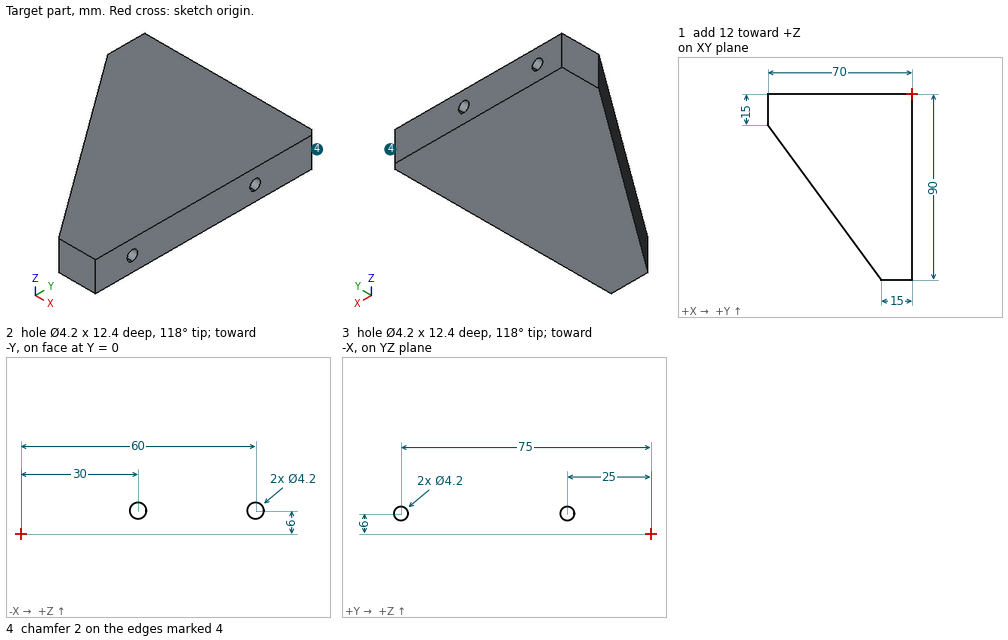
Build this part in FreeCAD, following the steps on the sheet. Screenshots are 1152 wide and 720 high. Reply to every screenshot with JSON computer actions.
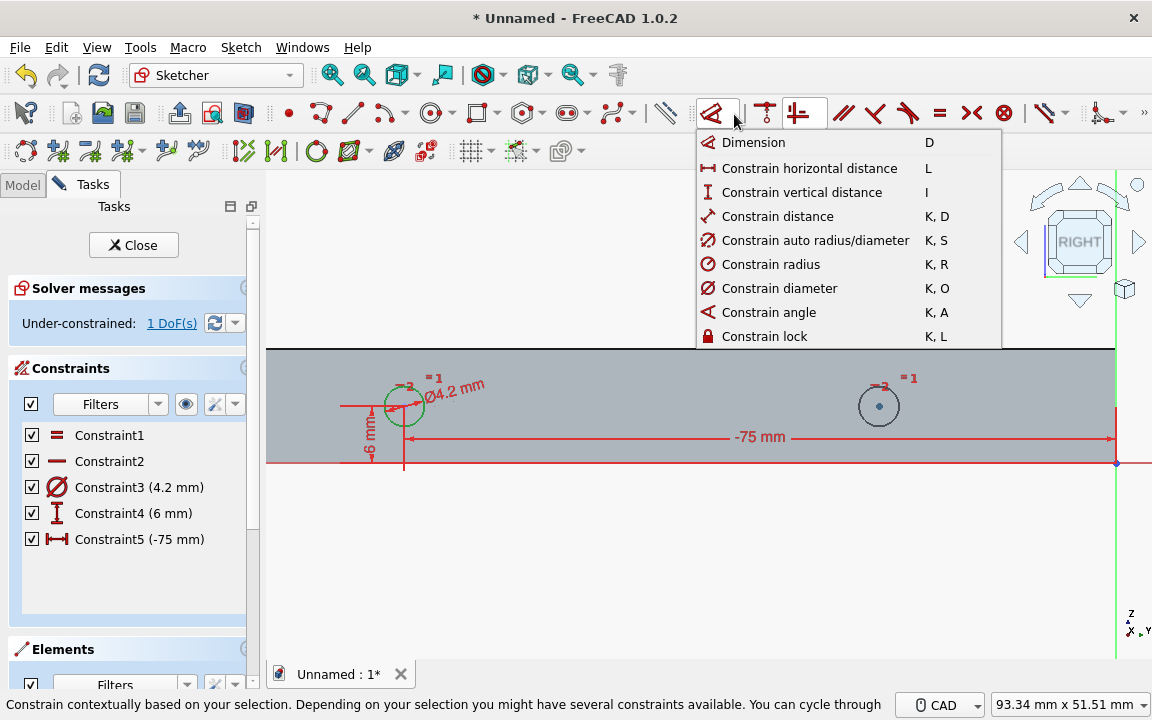
{"action": "left_click", "coordinate": [849, 168]}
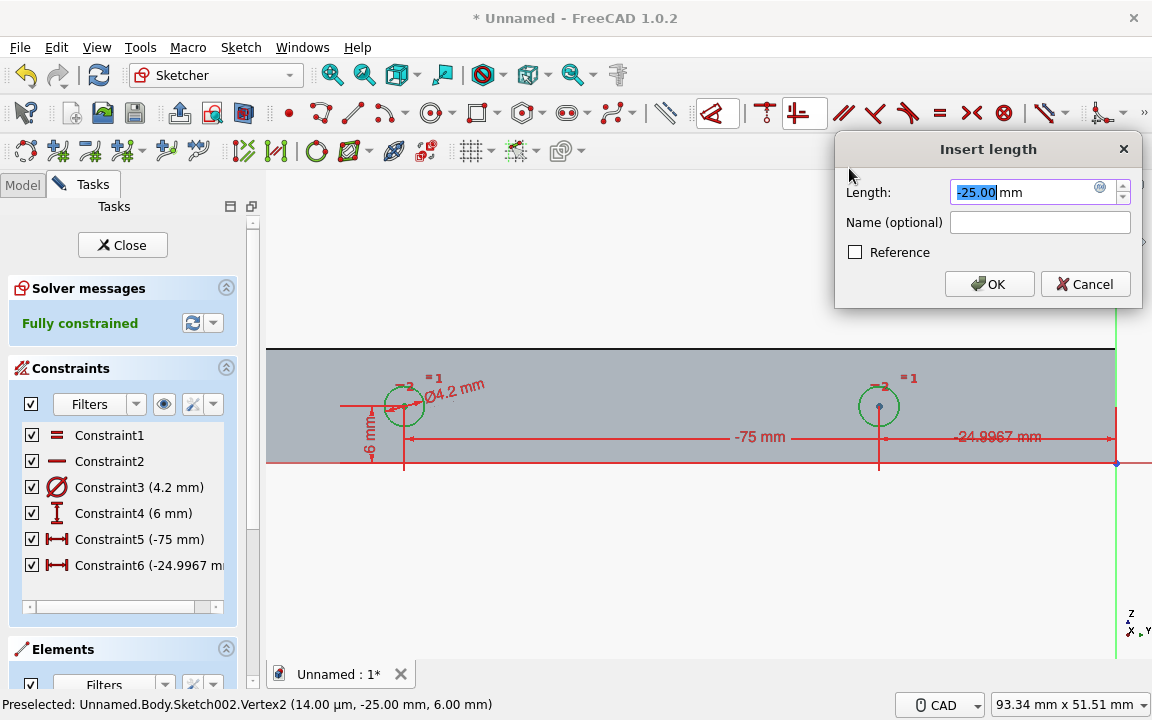
{"action": "type", "text": "-25"}
{"action": "key", "text": "Return"}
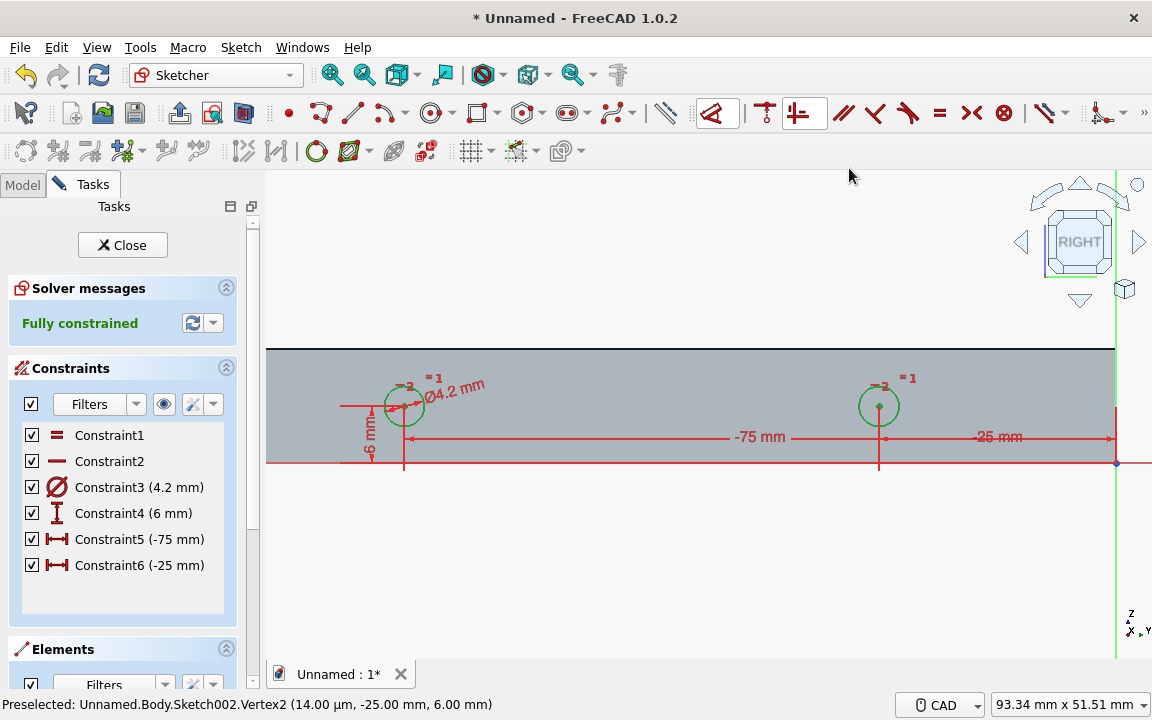
{"action": "left_click", "coordinate": [123, 245]}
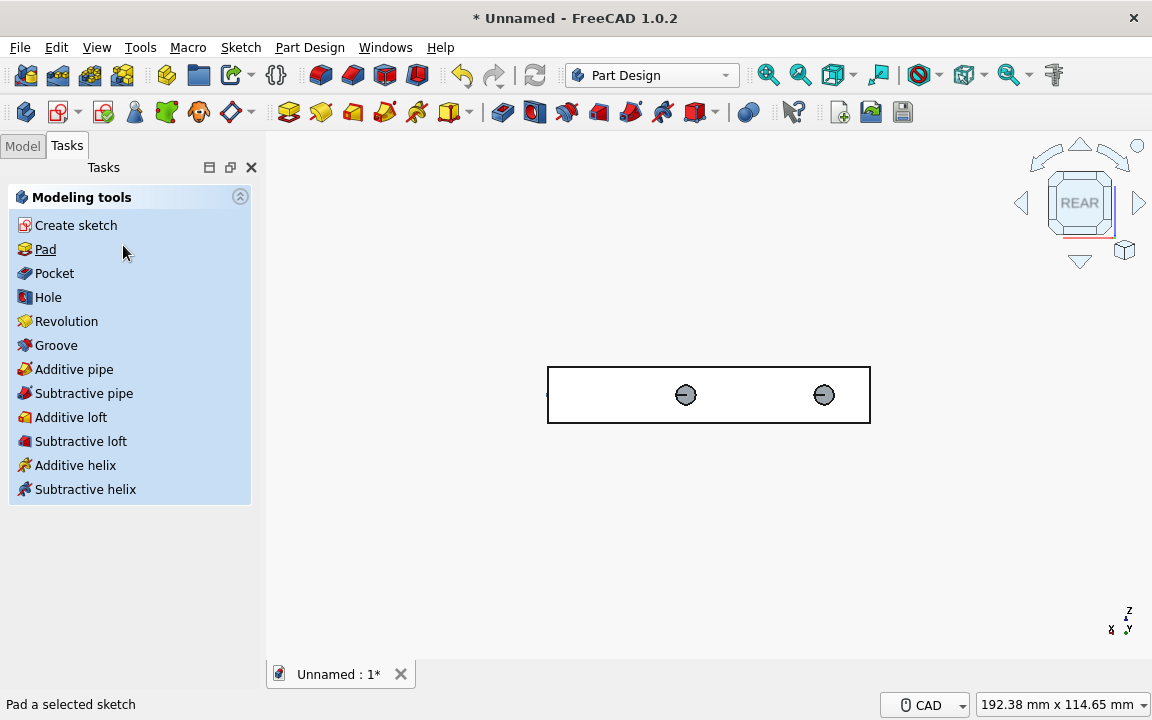
{"action": "left_click", "coordinate": [536, 112]}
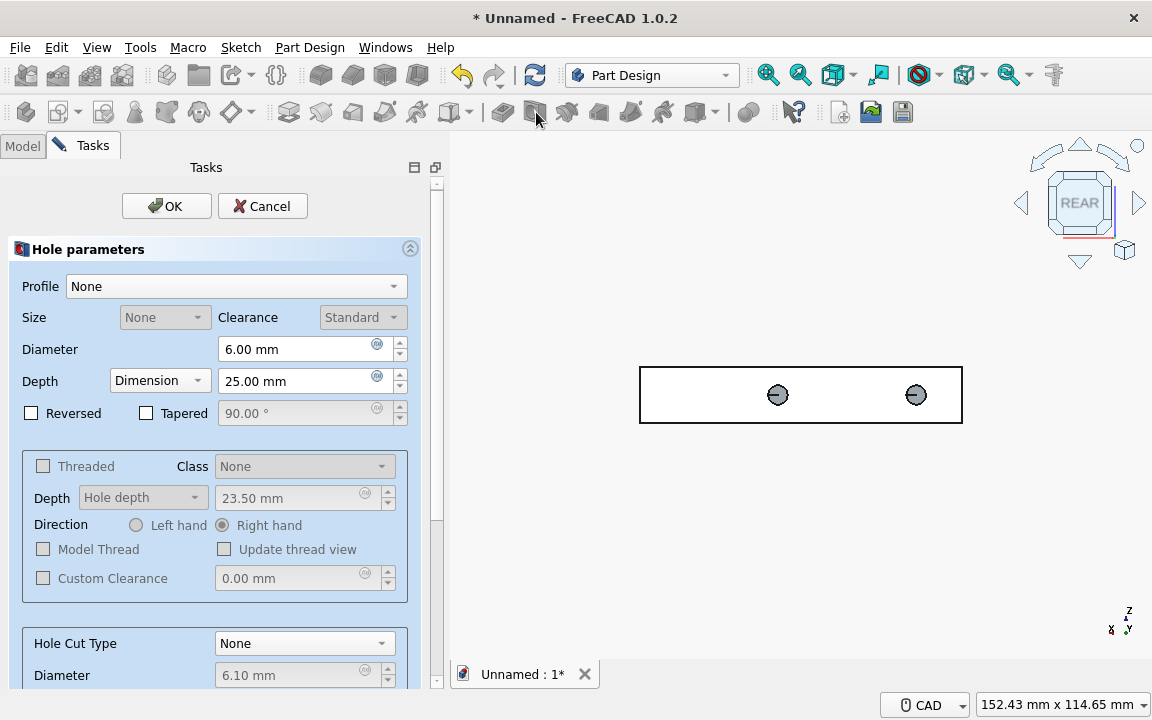
{"action": "triple_click", "coordinate": [305, 349]}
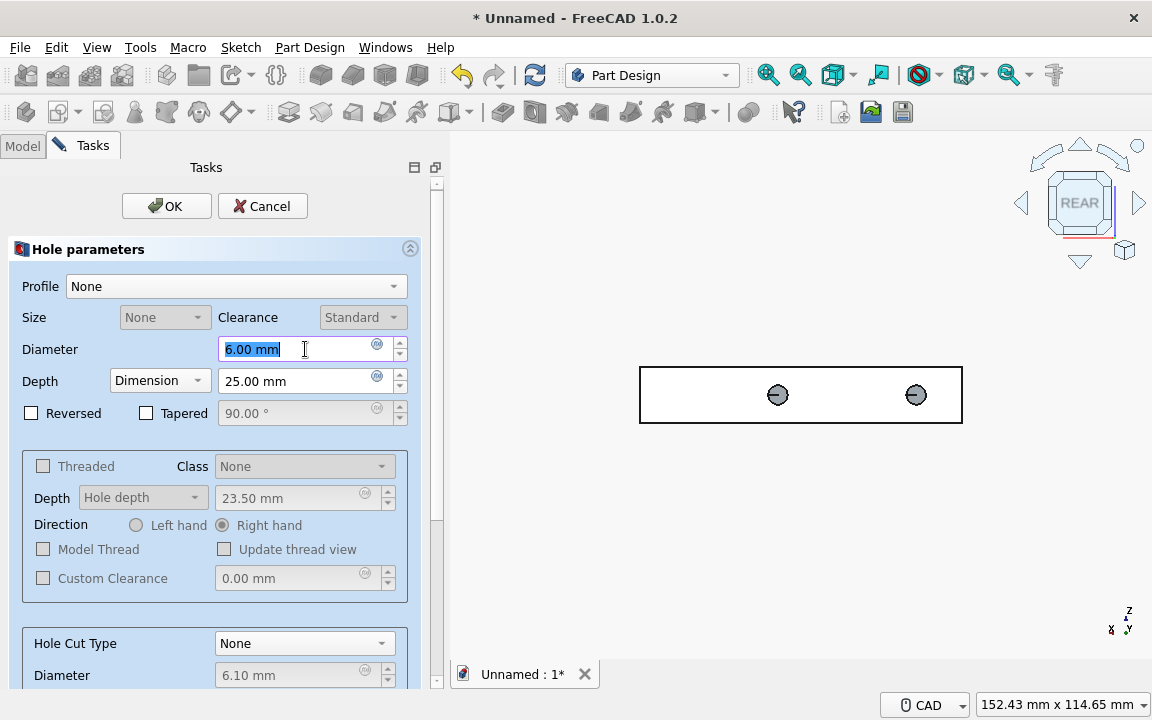
{"action": "type", "text": "4.2"}
{"action": "key", "text": "Tab"}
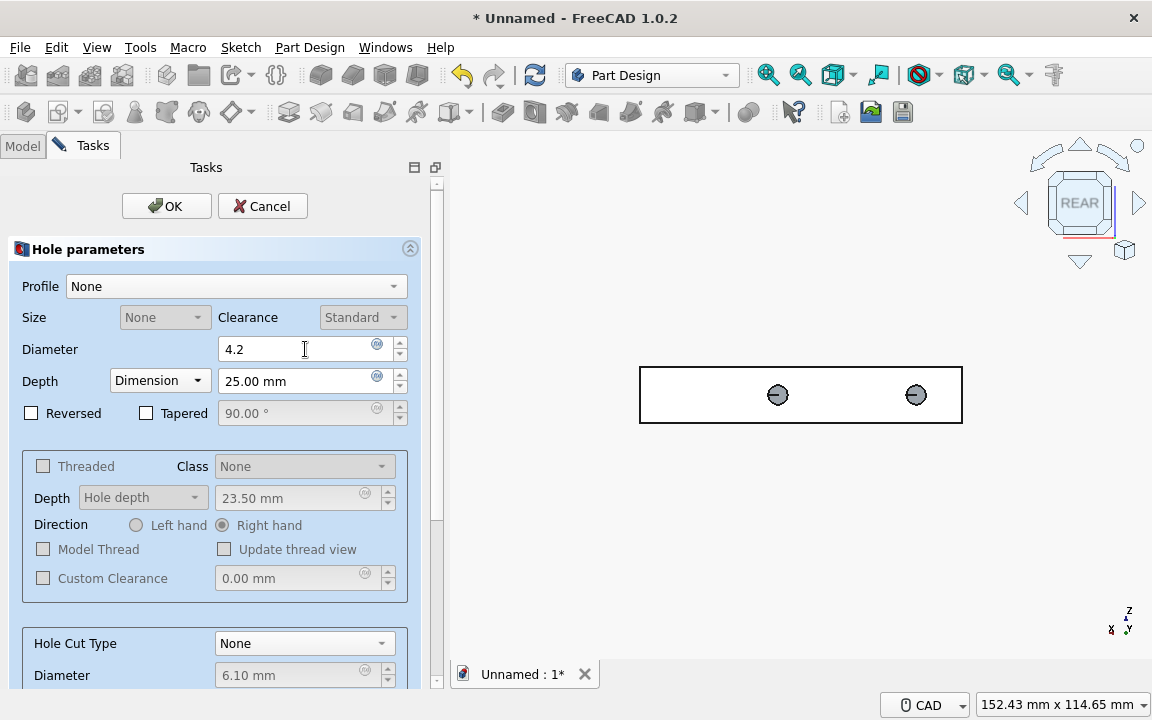
{"action": "triple_click", "coordinate": [305, 381]}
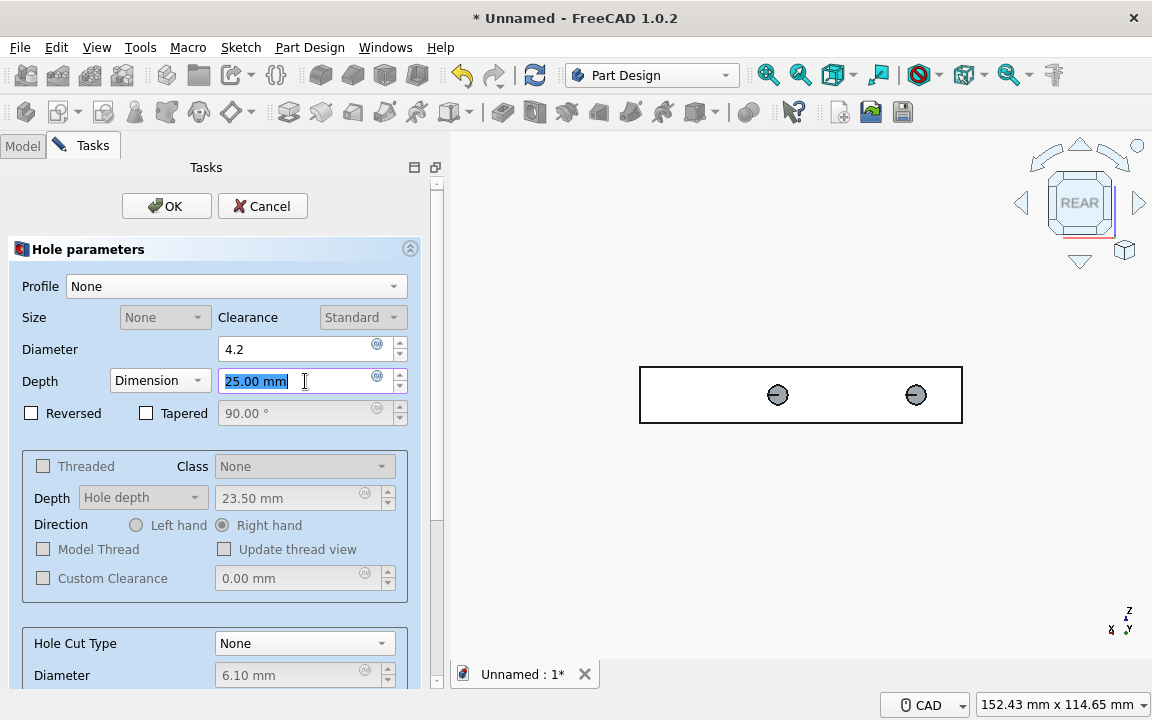
{"action": "type", "text": "12.4"}
{"action": "key", "text": "Tab"}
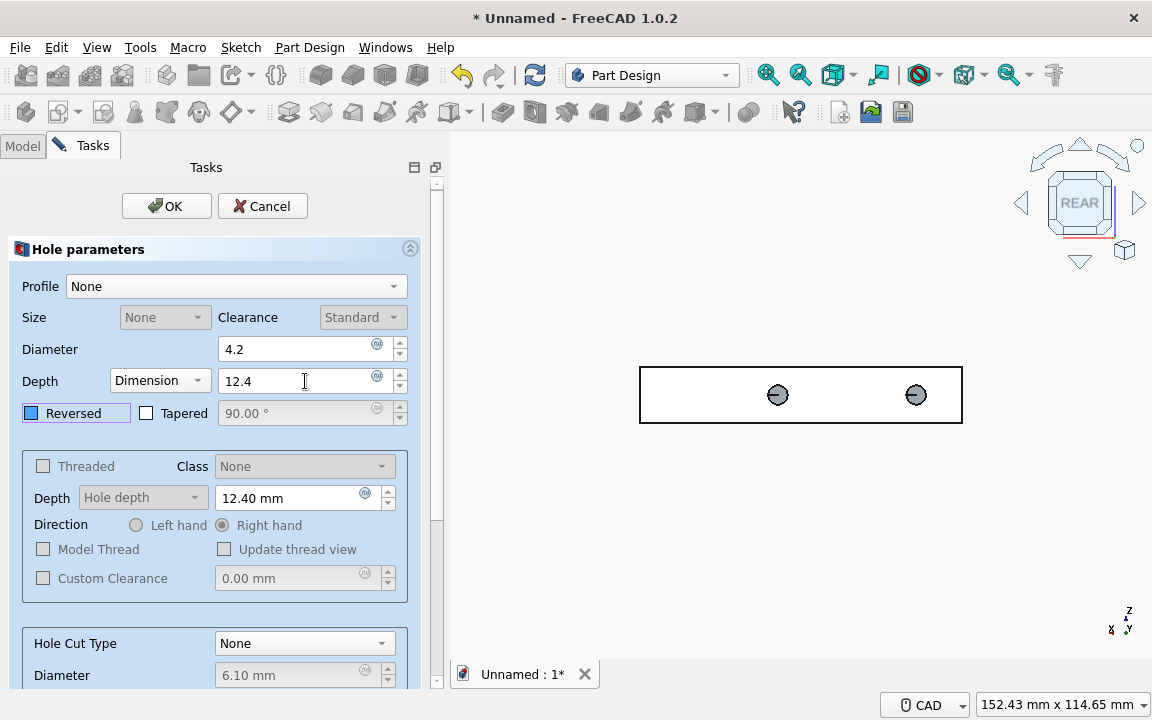
{"action": "left_click", "coordinate": [167, 206]}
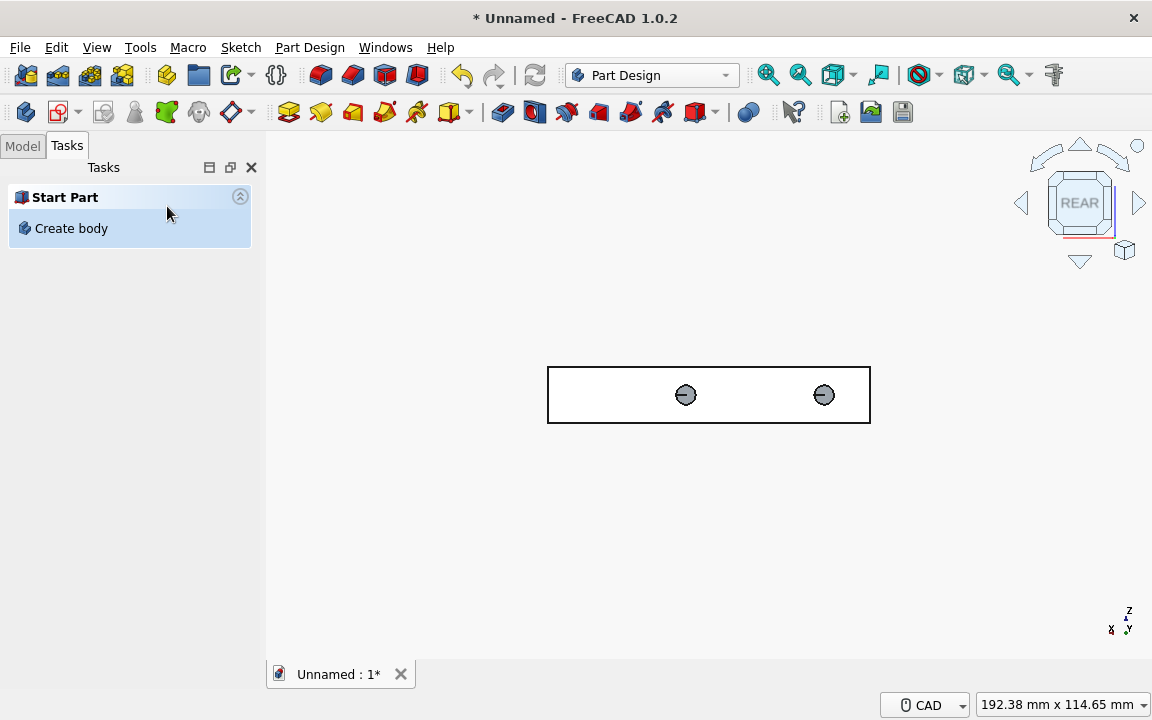
{"action": "key", "text": "v f"}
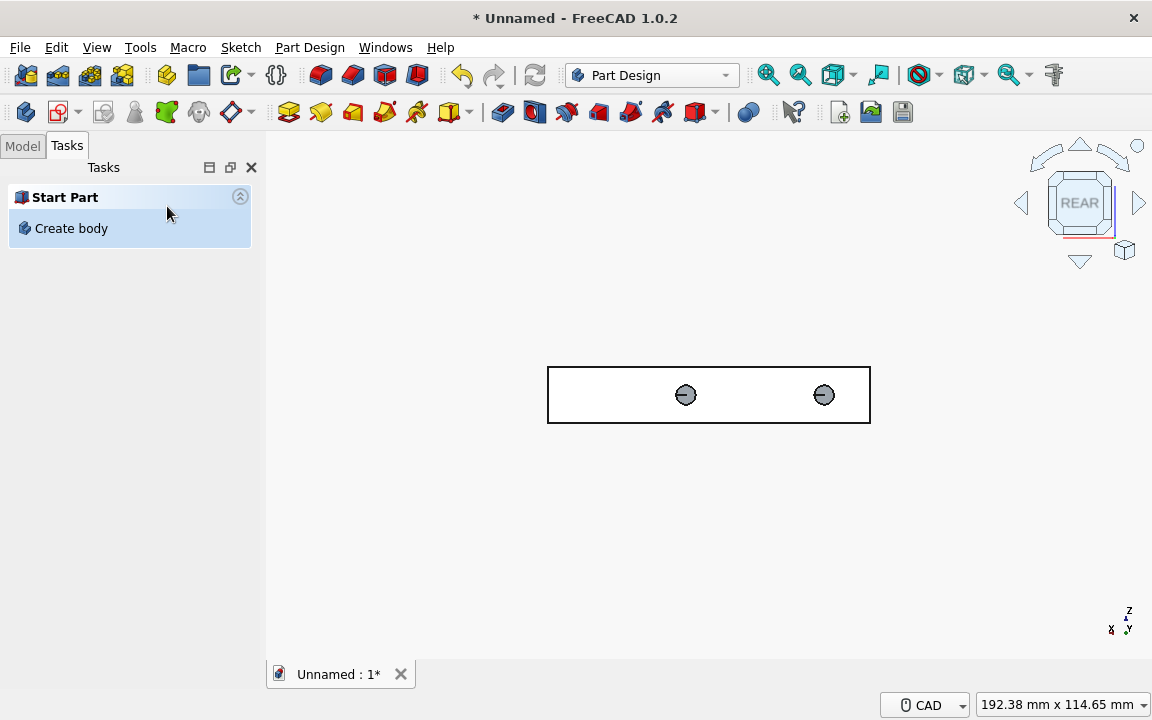
{"action": "key", "text": "0"}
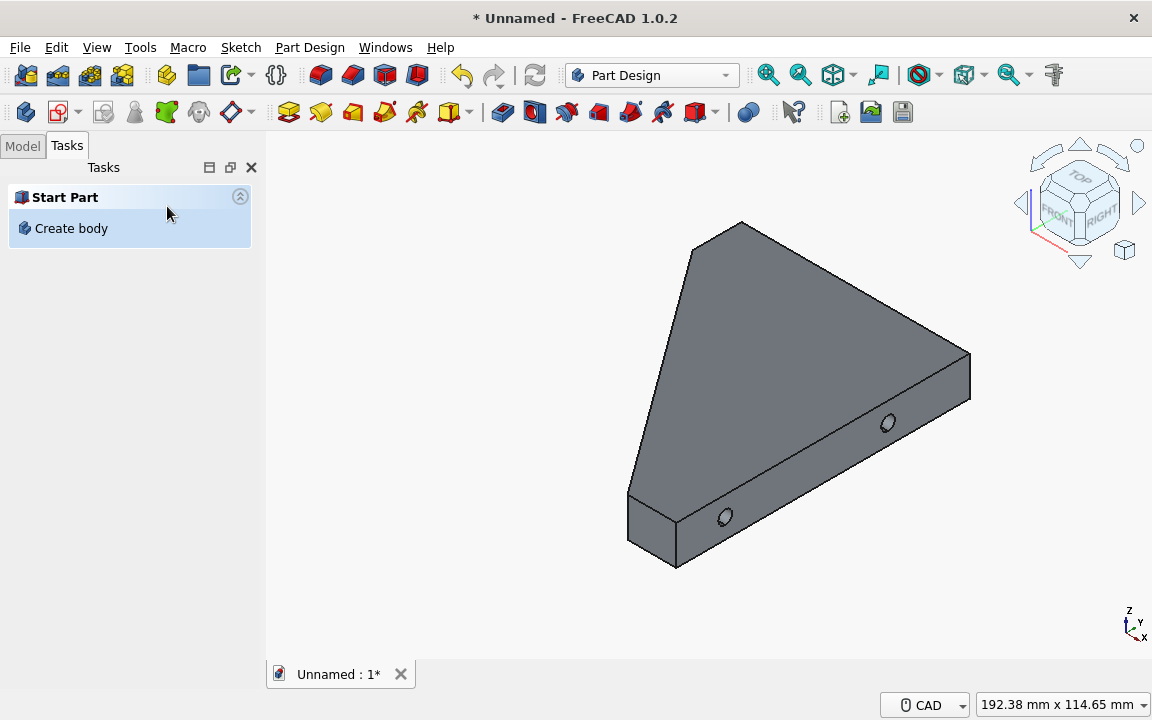
{"action": "key", "text": "2"}